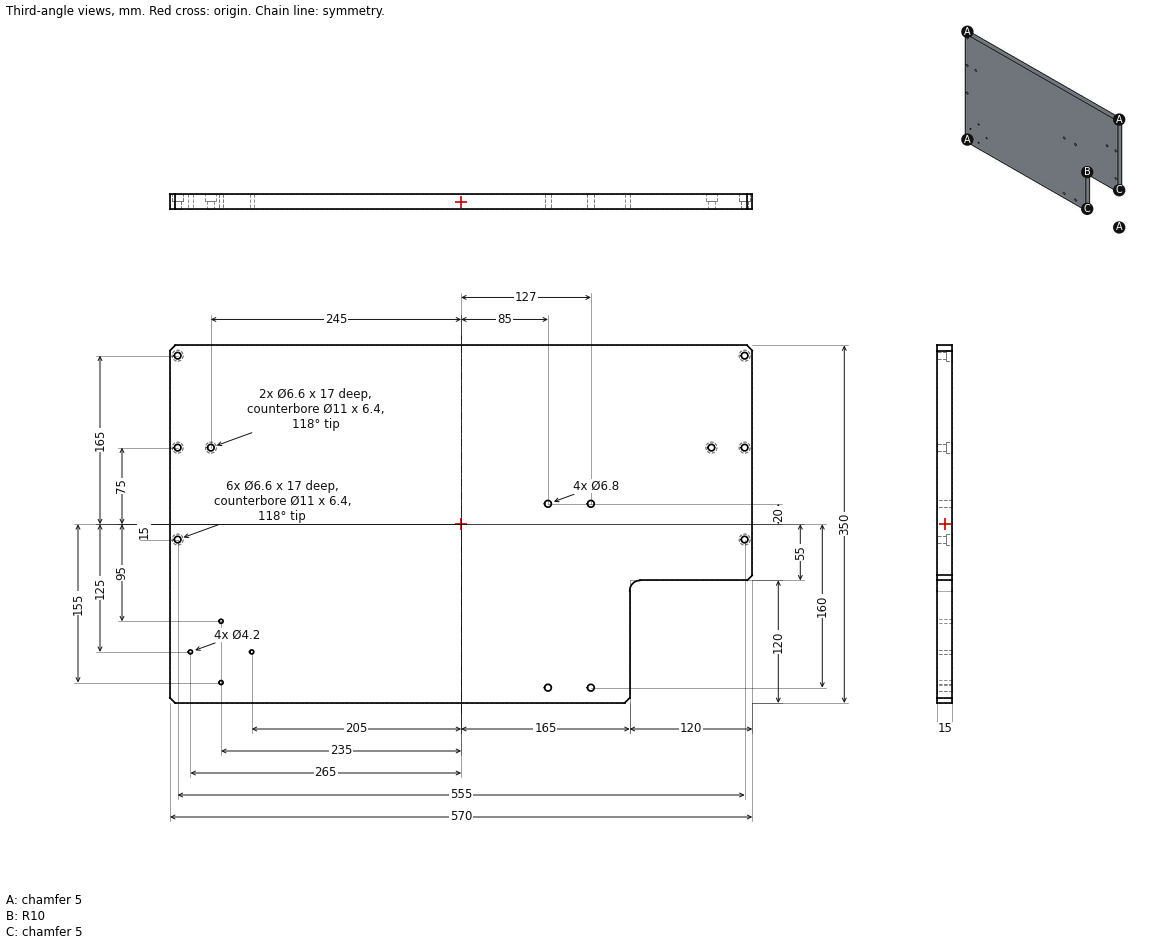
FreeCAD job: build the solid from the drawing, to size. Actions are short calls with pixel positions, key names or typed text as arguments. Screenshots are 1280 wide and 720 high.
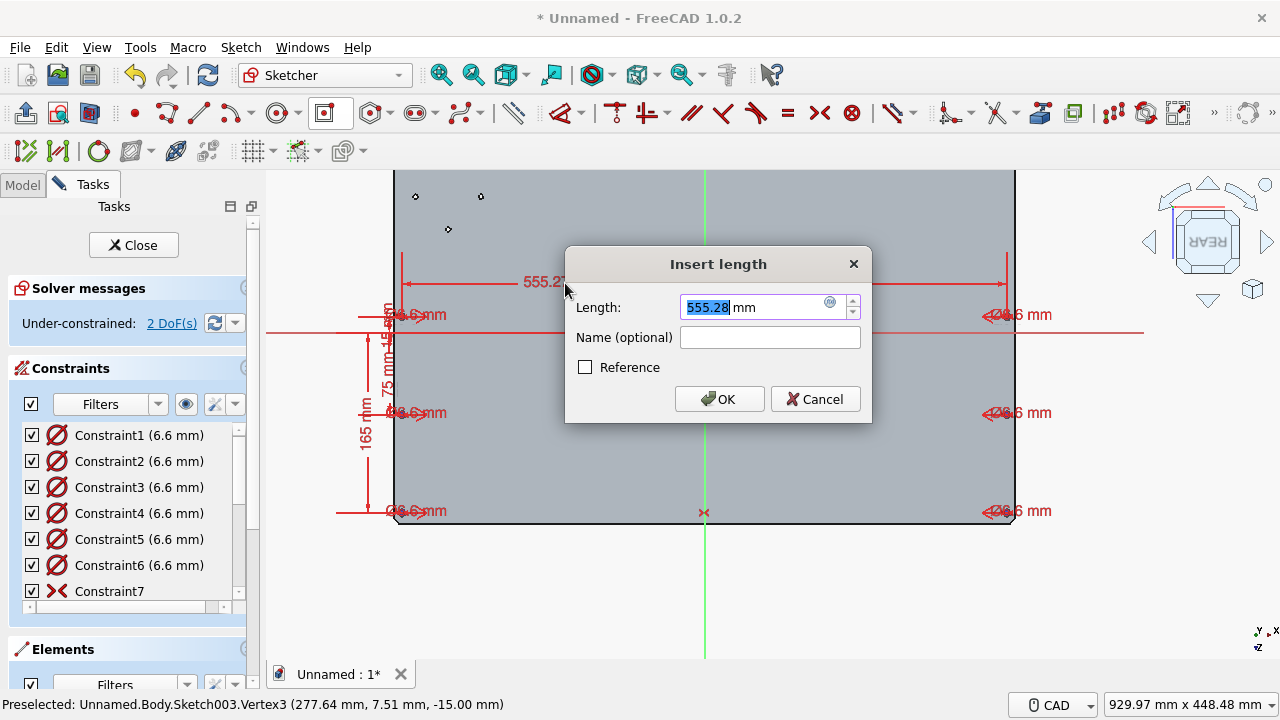
text(555)
key(Return)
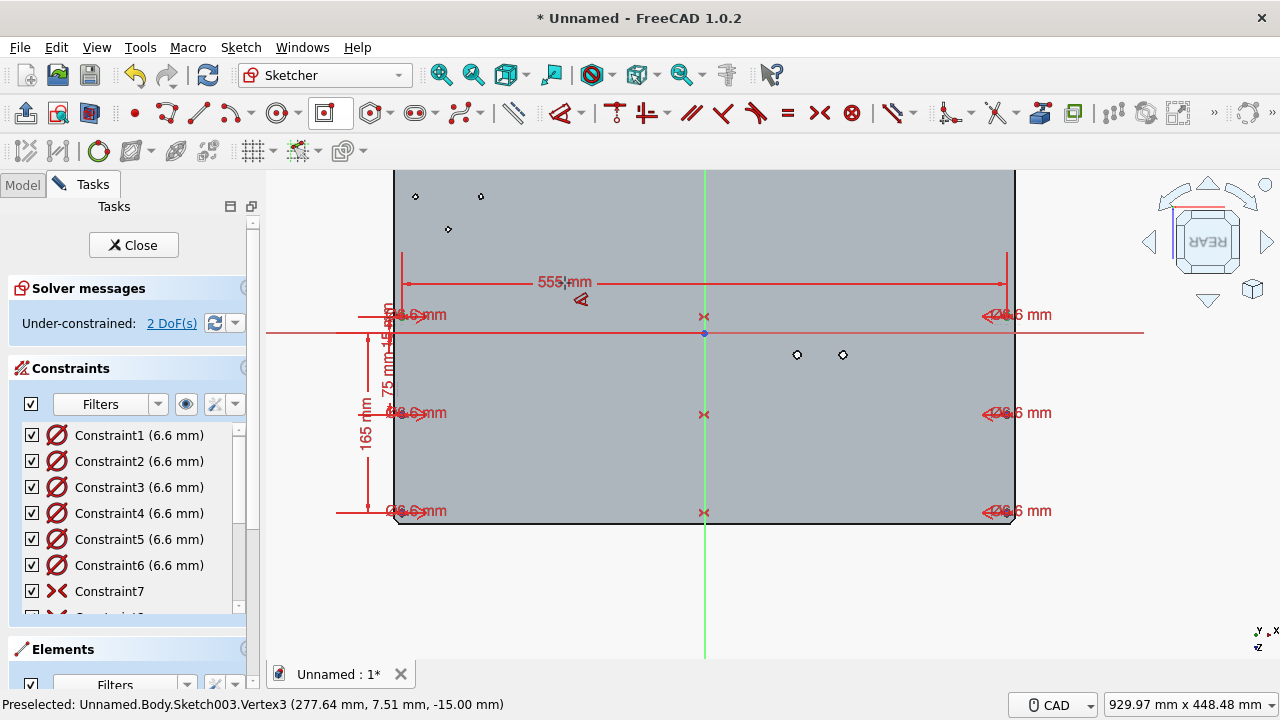
click(402, 513)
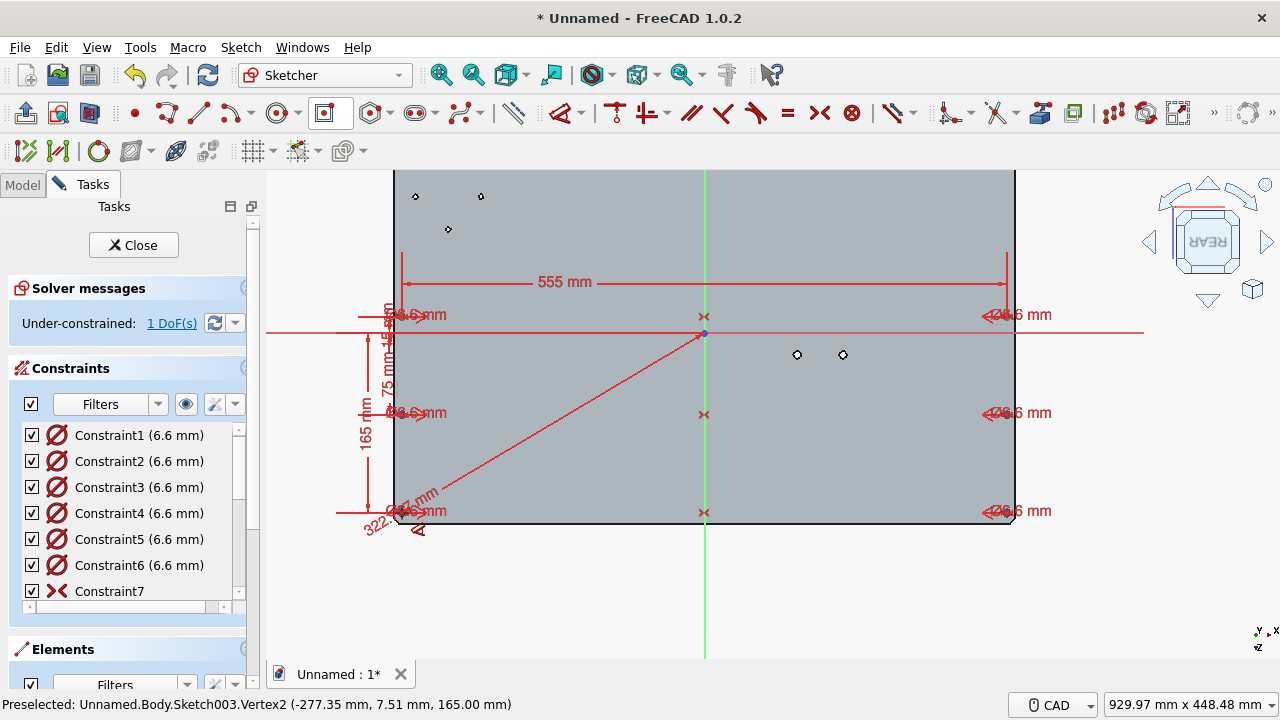
click(1007, 317)
click(565, 547)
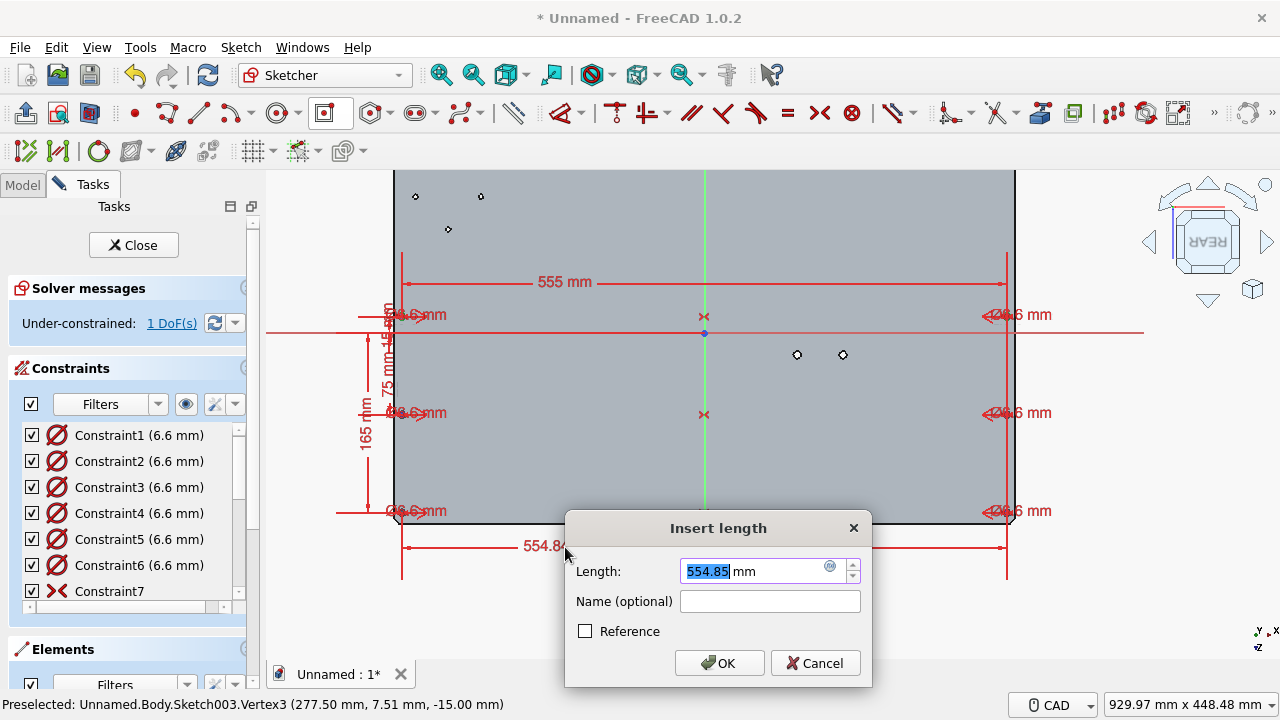
text(555)
key(Return)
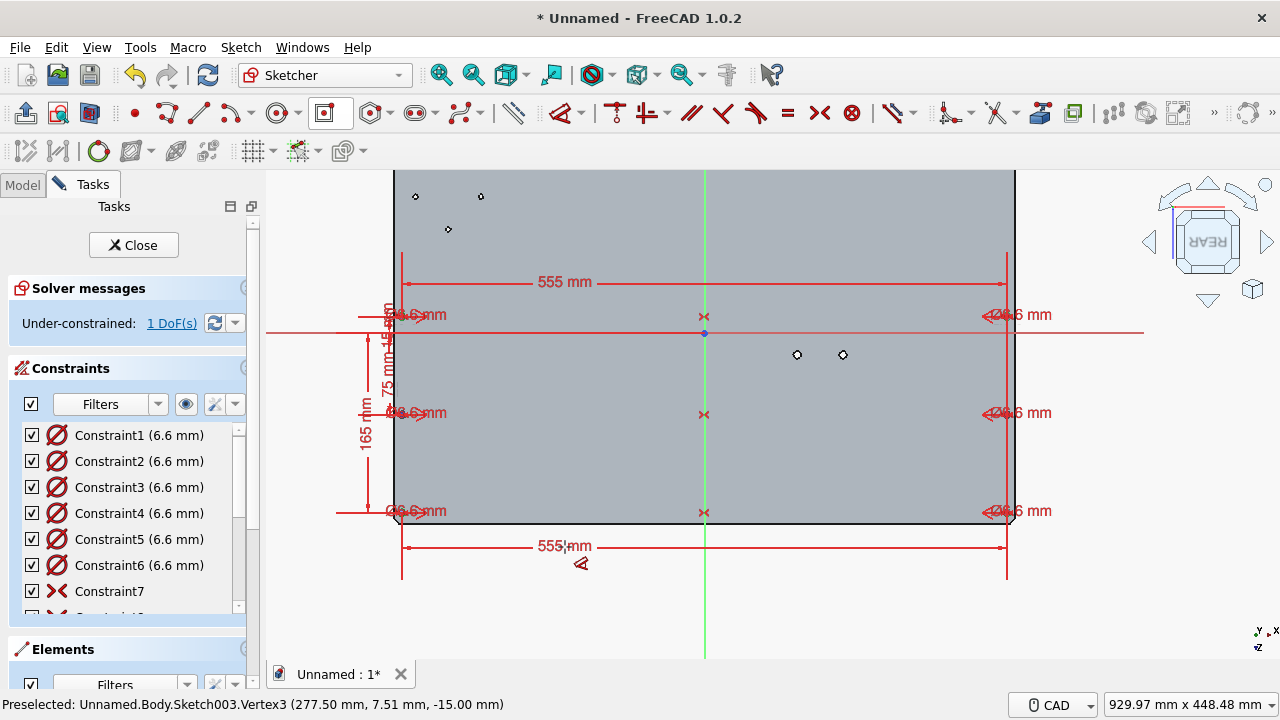
click(1007, 317)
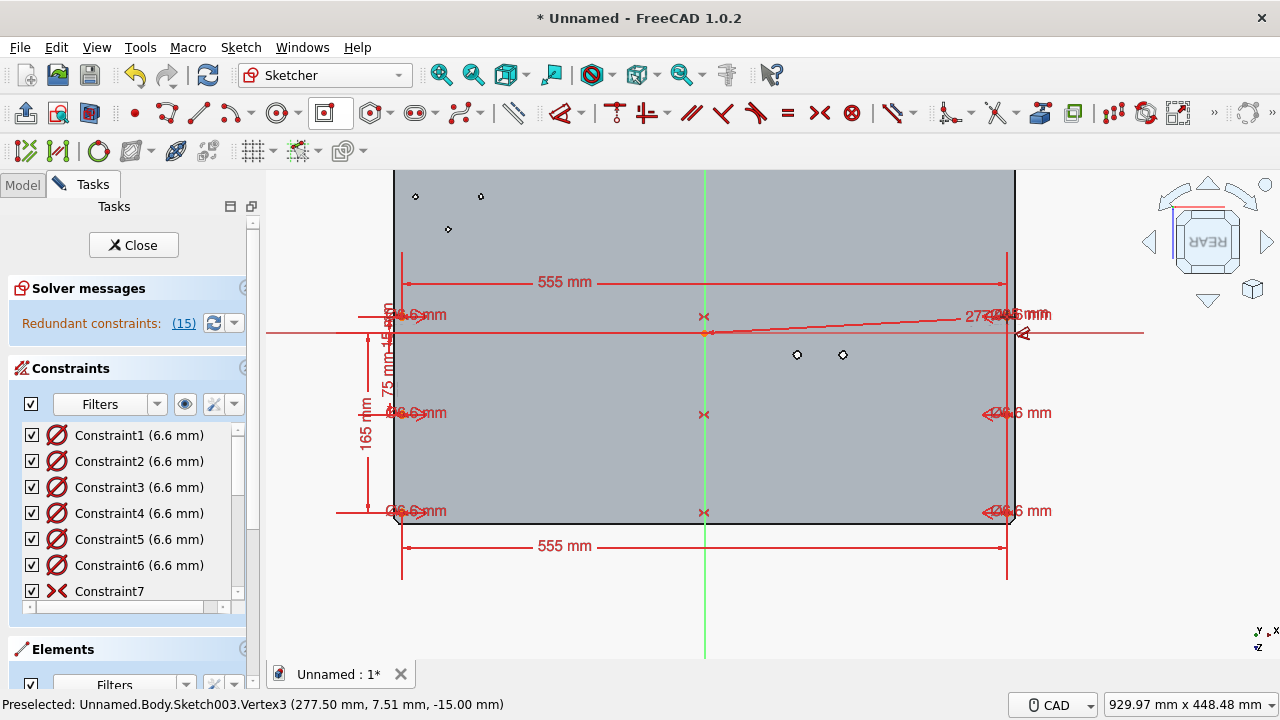
click(402, 415)
click(844, 283)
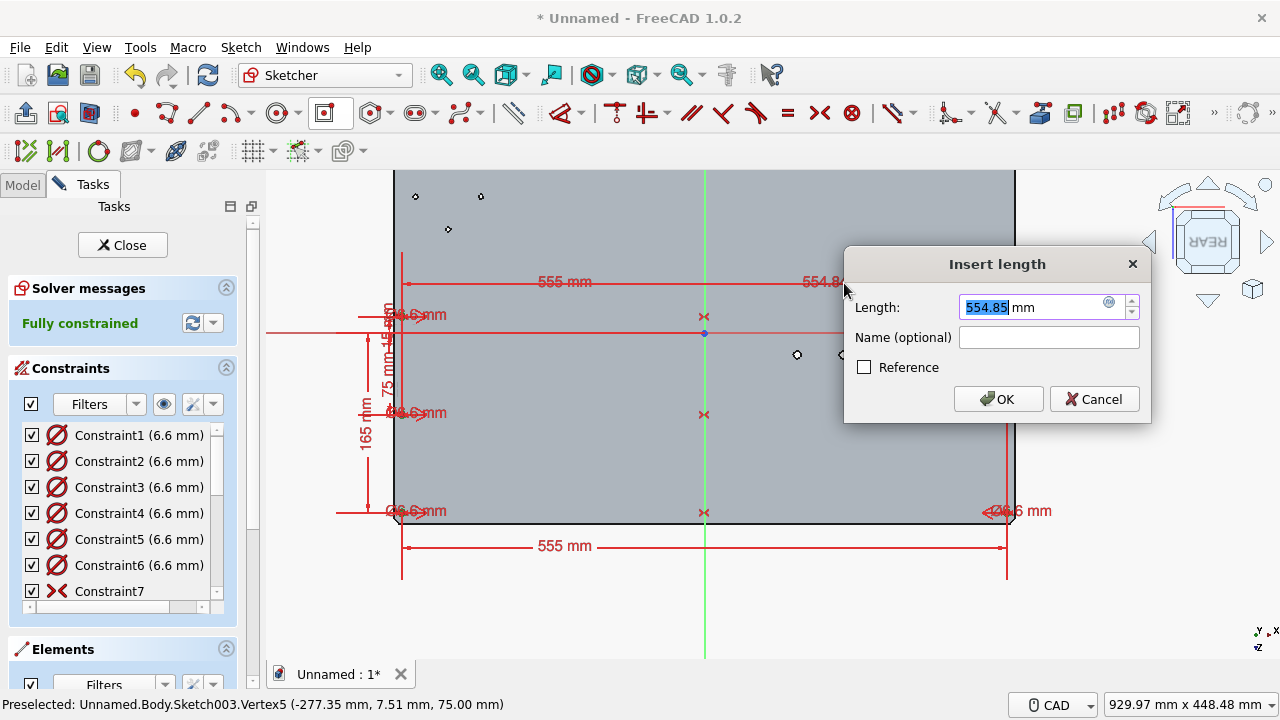
text(555)
key(Return)
key(Escape)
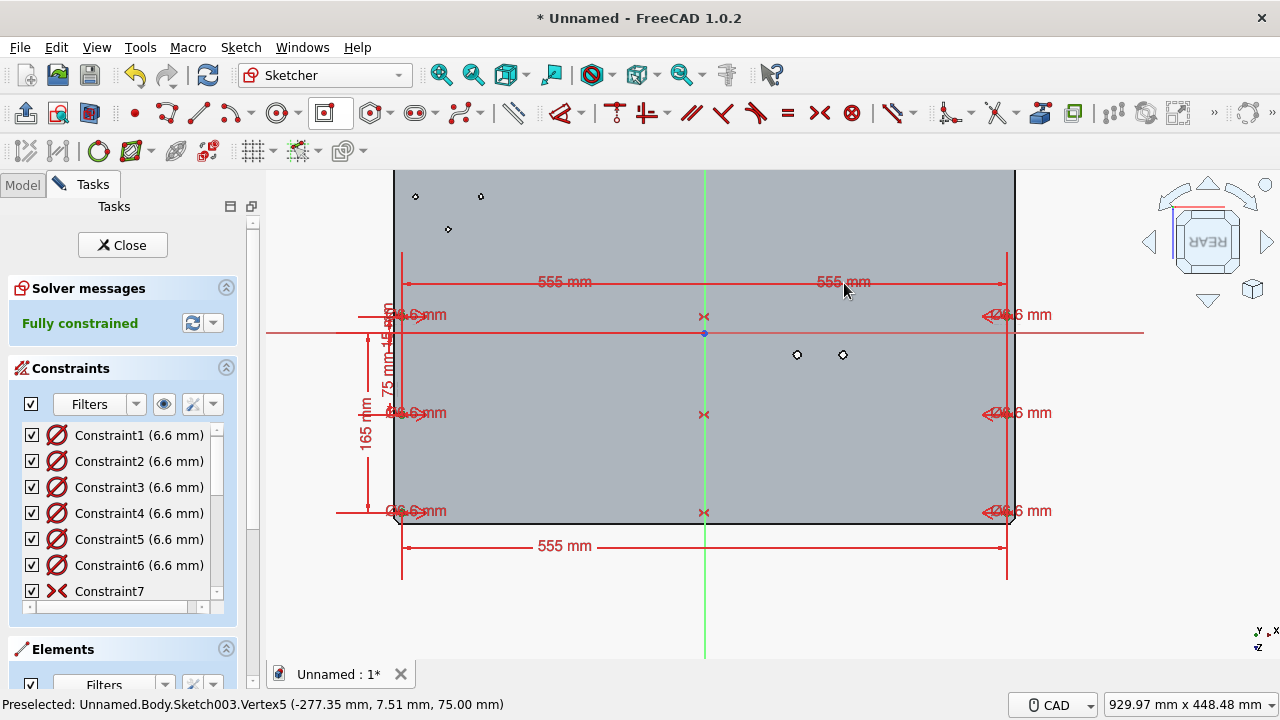
click(123, 245)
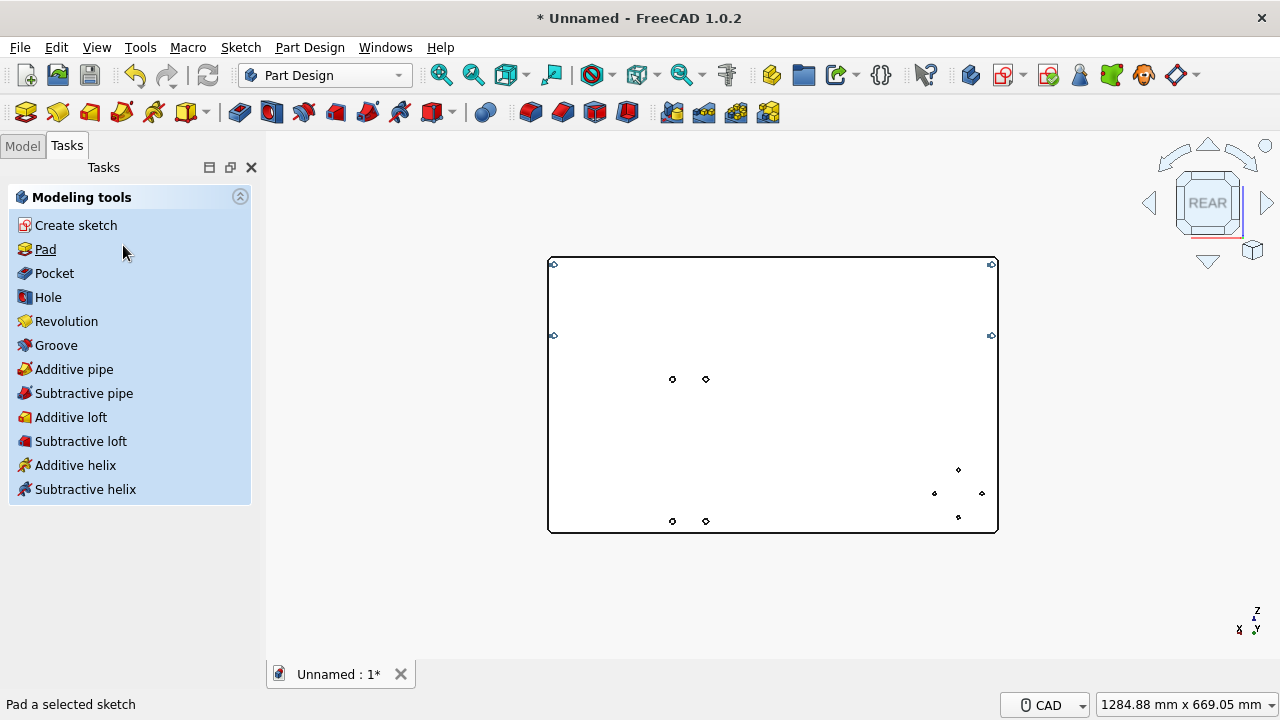
click(272, 112)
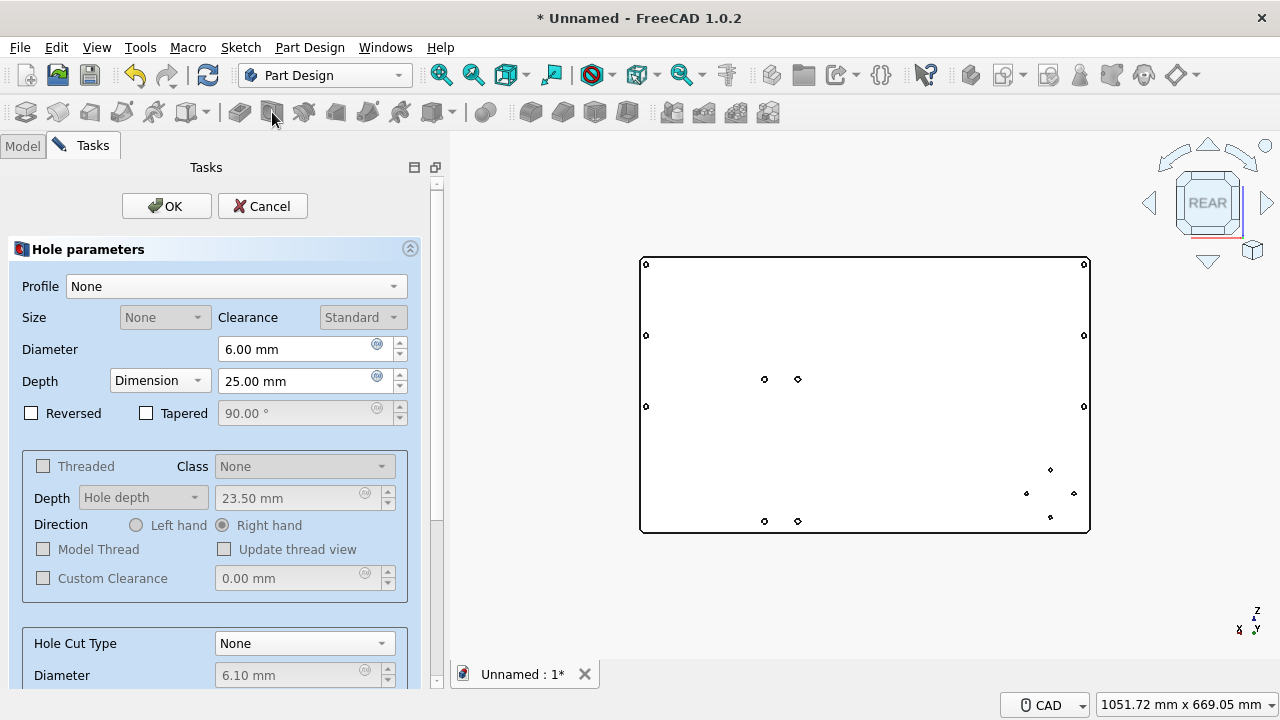
triple_click(305, 349)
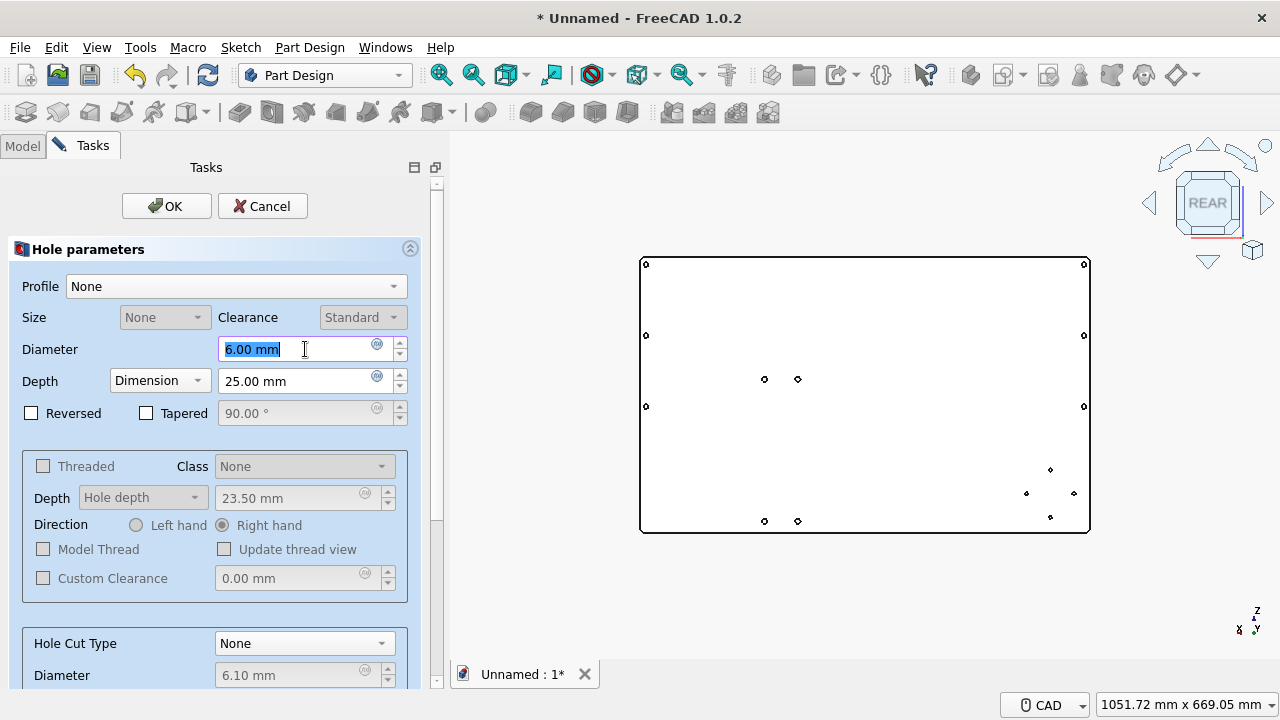
text(6.6)
key(Tab)